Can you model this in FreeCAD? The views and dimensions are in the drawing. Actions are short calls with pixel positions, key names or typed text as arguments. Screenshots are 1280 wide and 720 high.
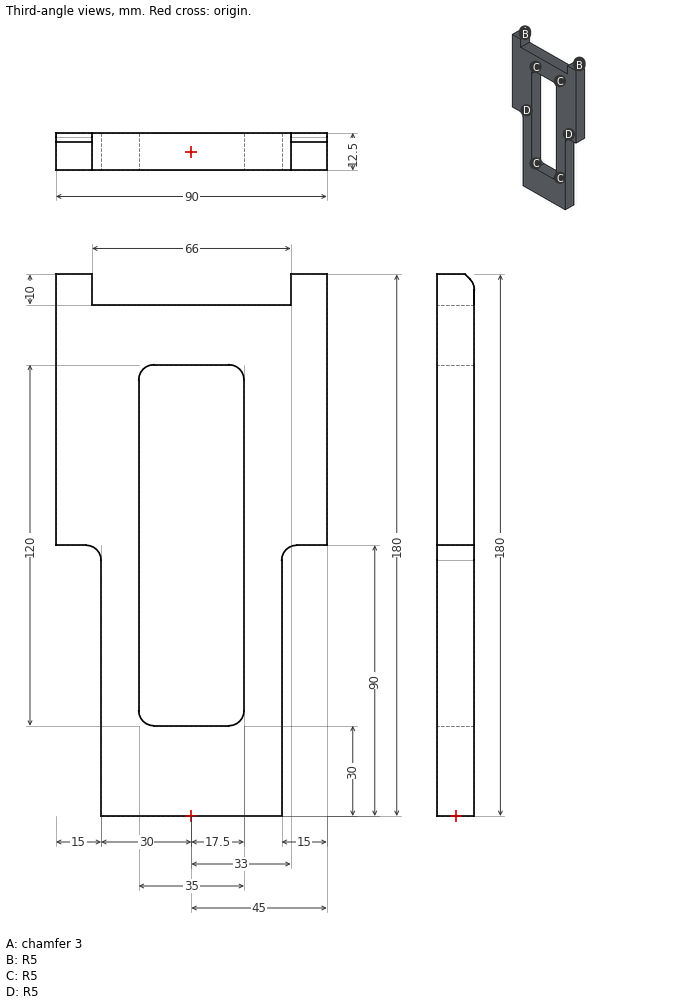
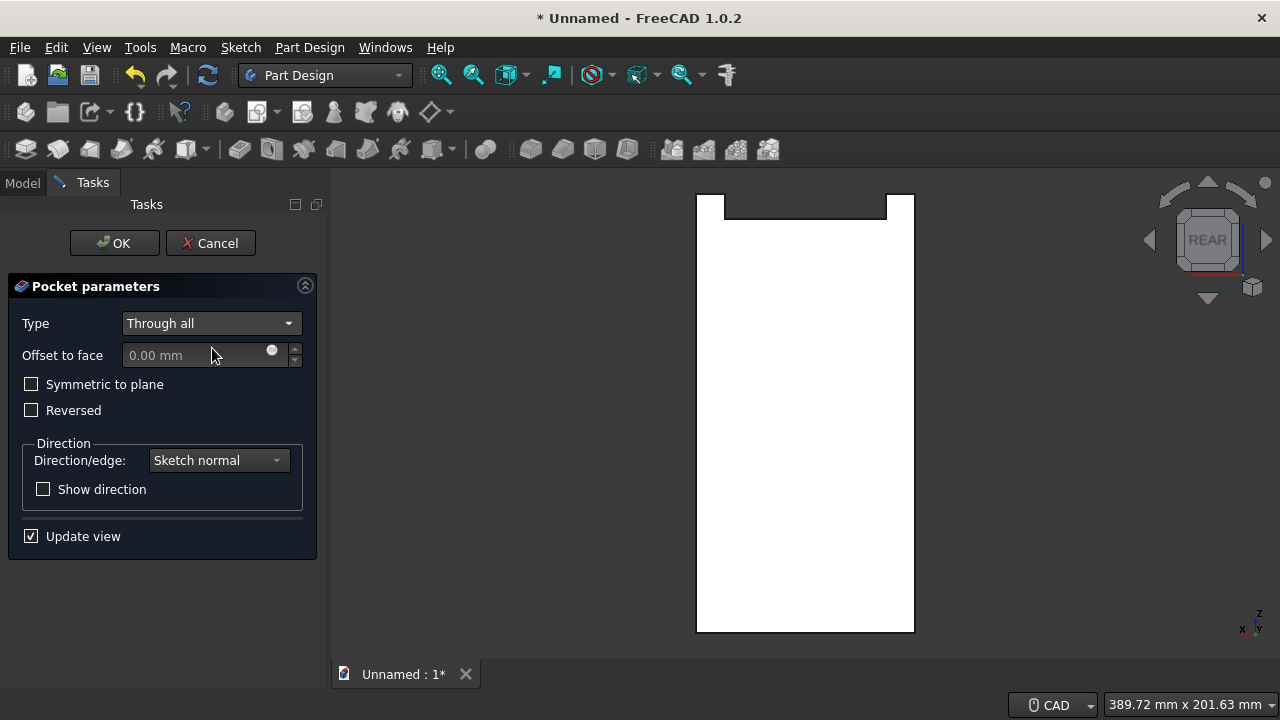
click(115, 243)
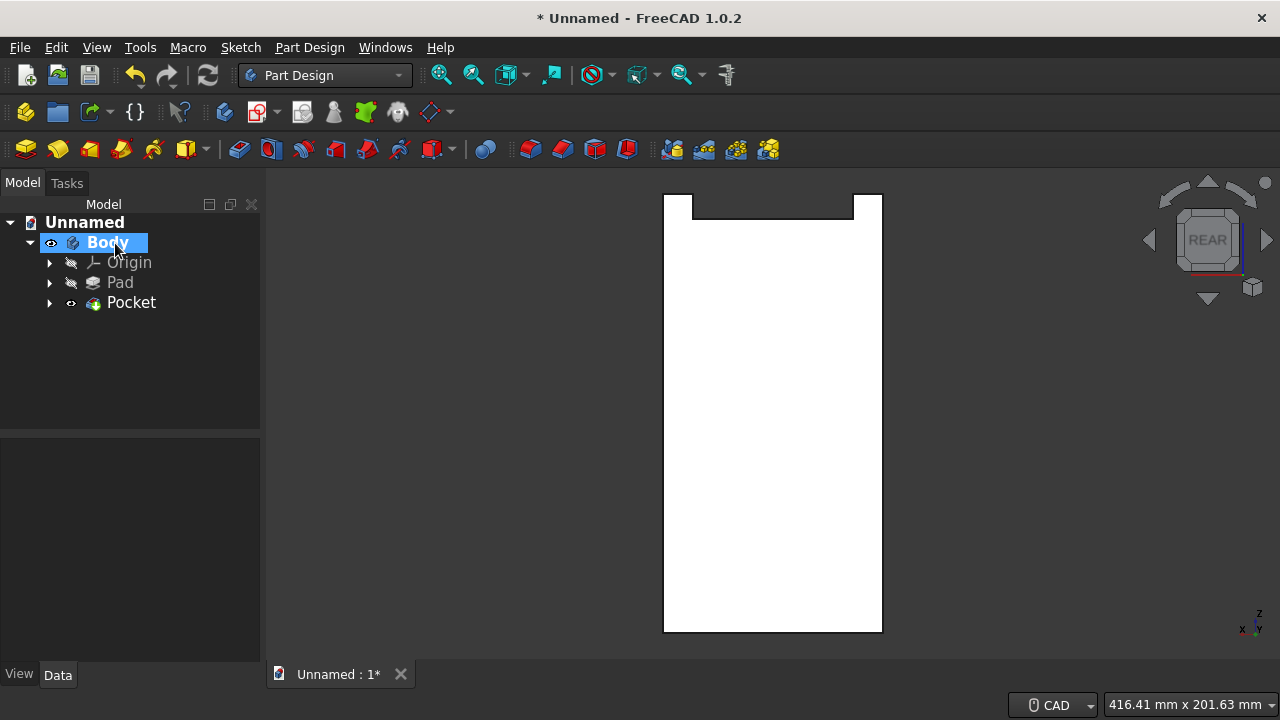
key(0)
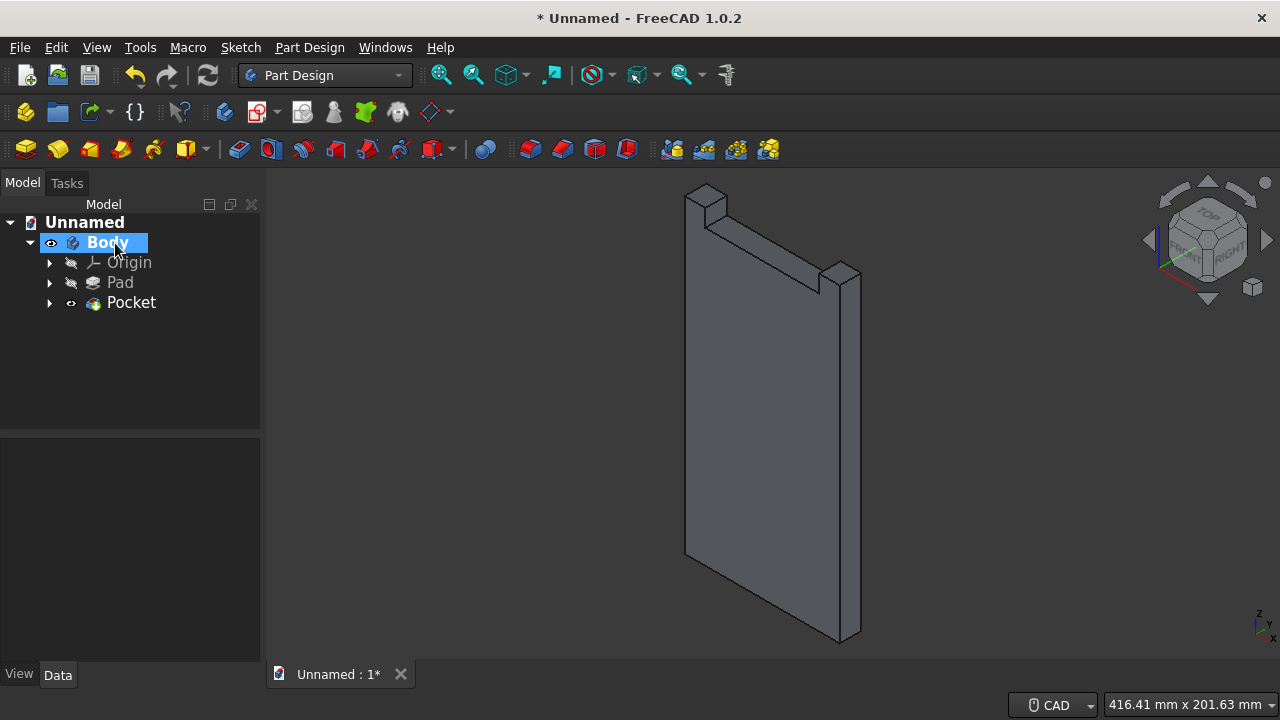
key(2)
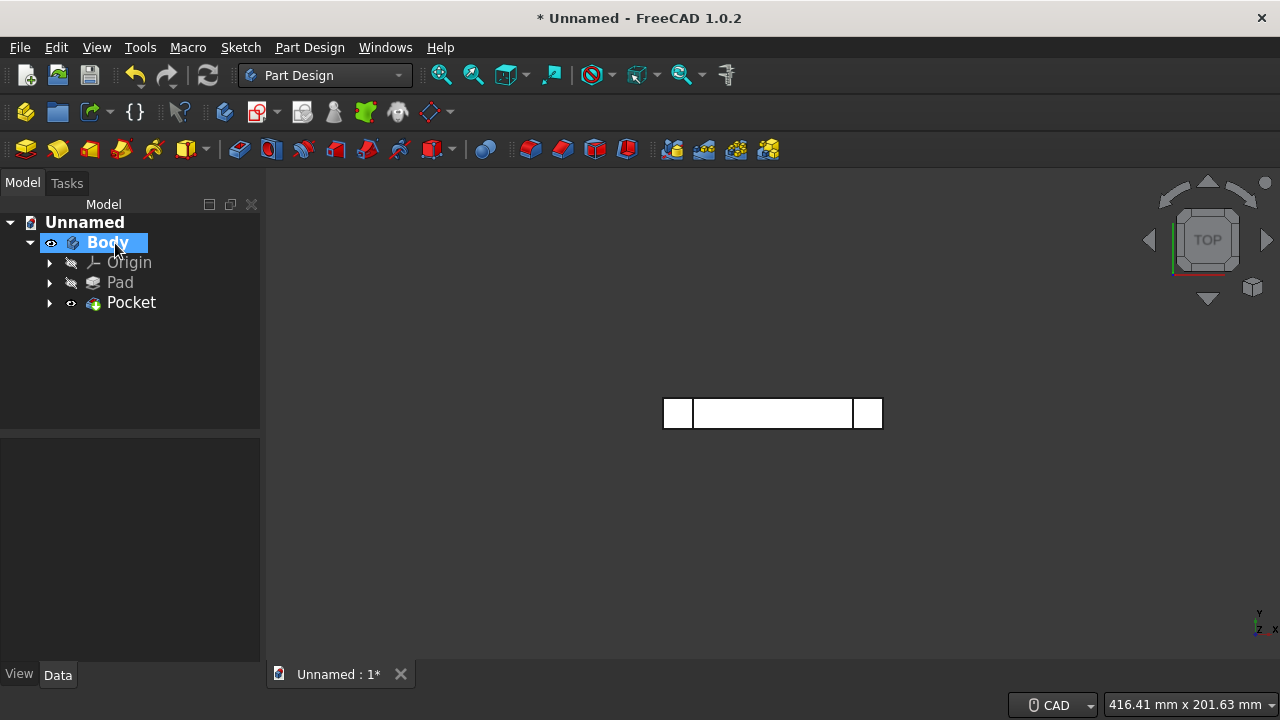
click(442, 76)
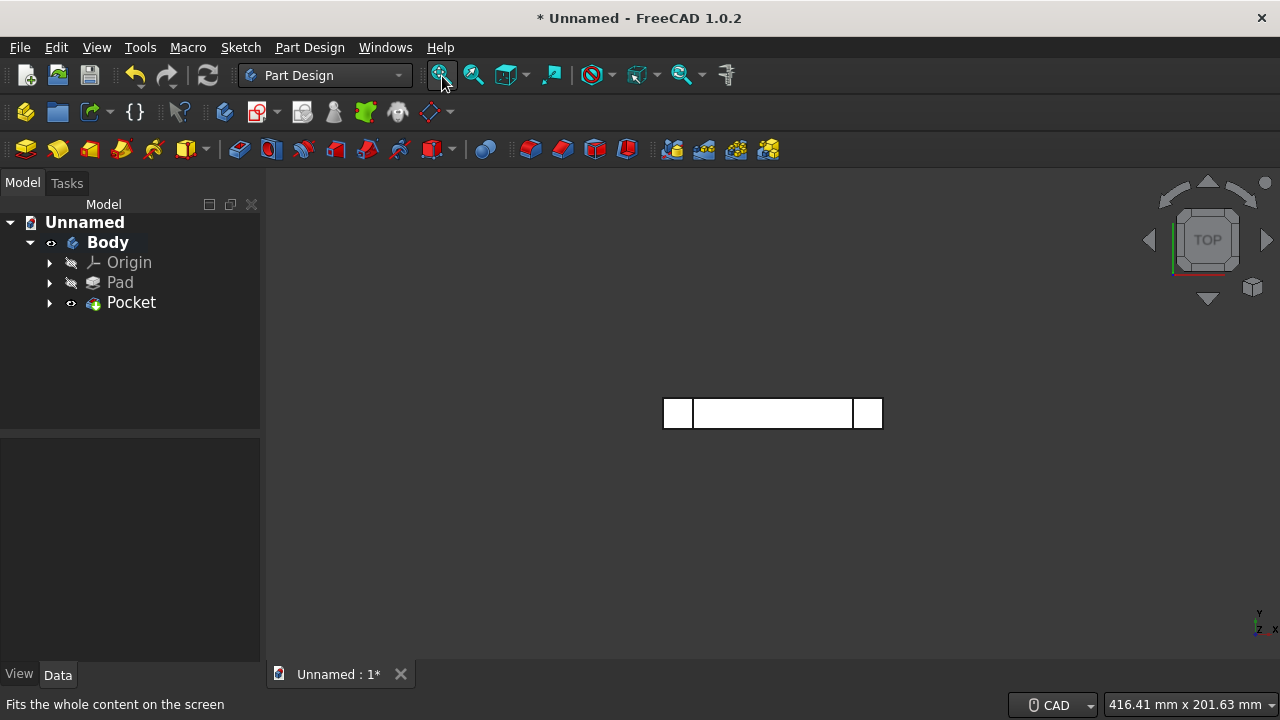
click(868, 397)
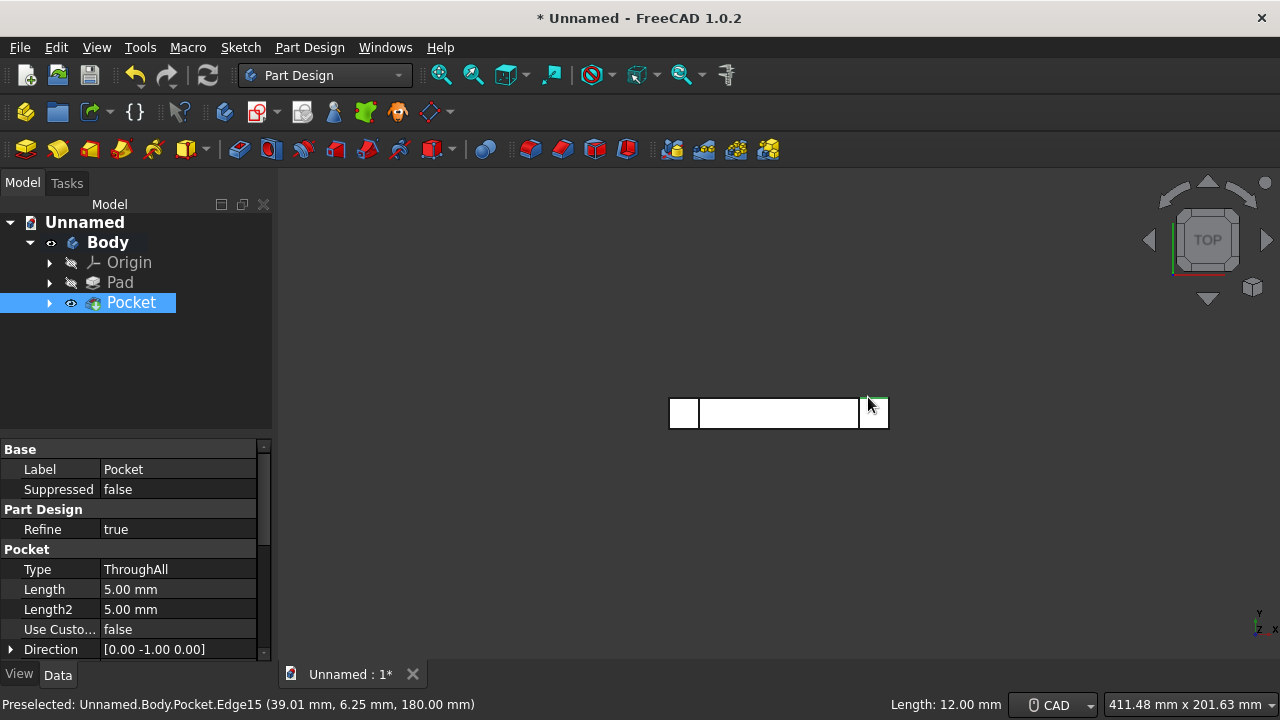
click(684, 397, ctrl)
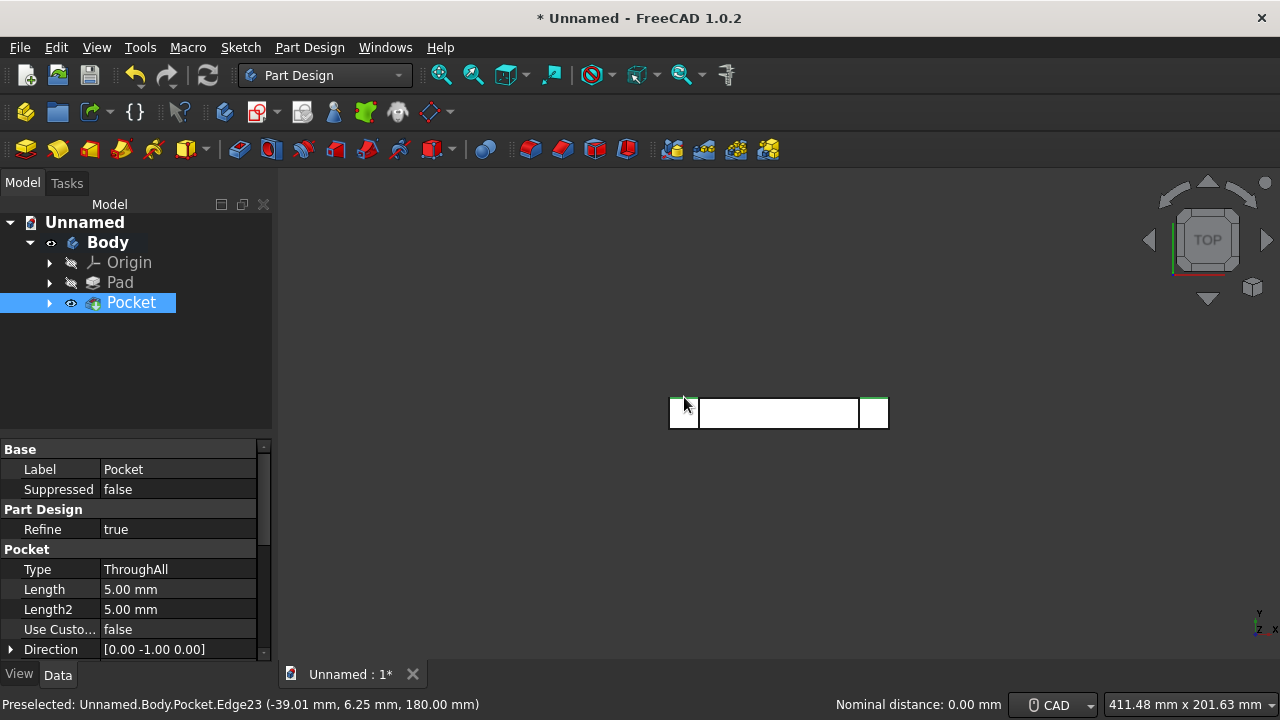
click(564, 150)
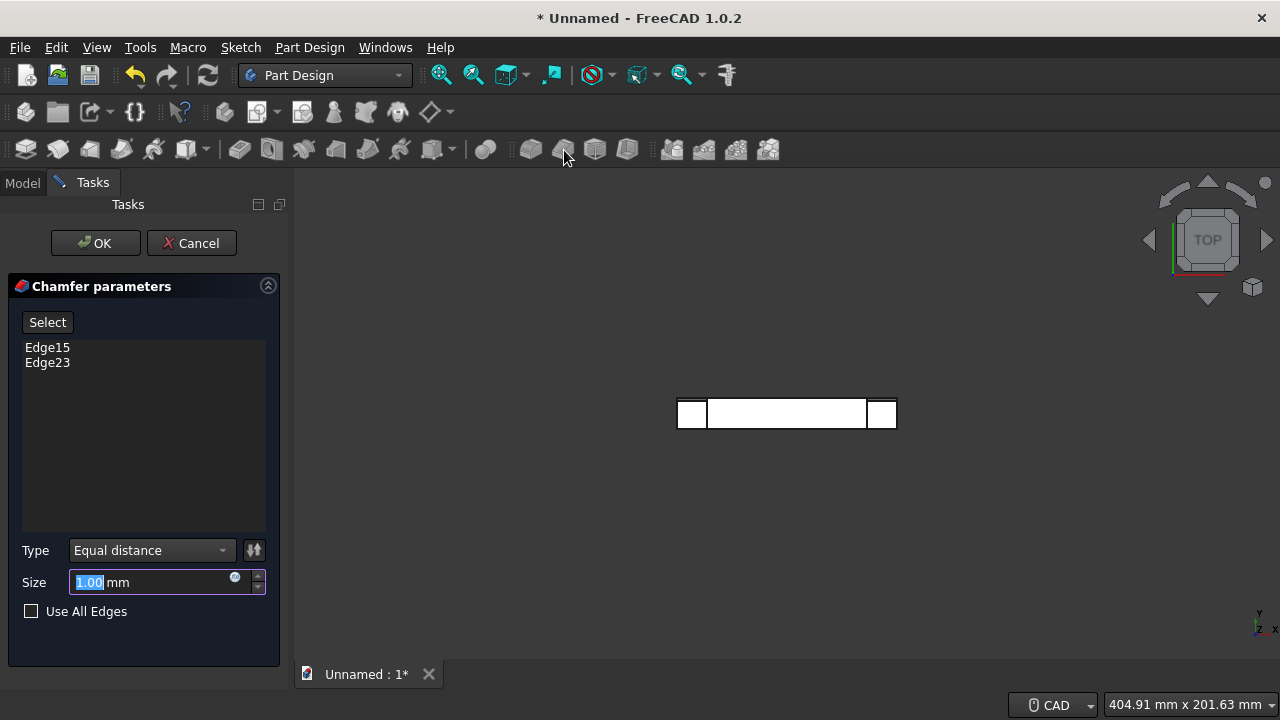
text(3)
key(Tab)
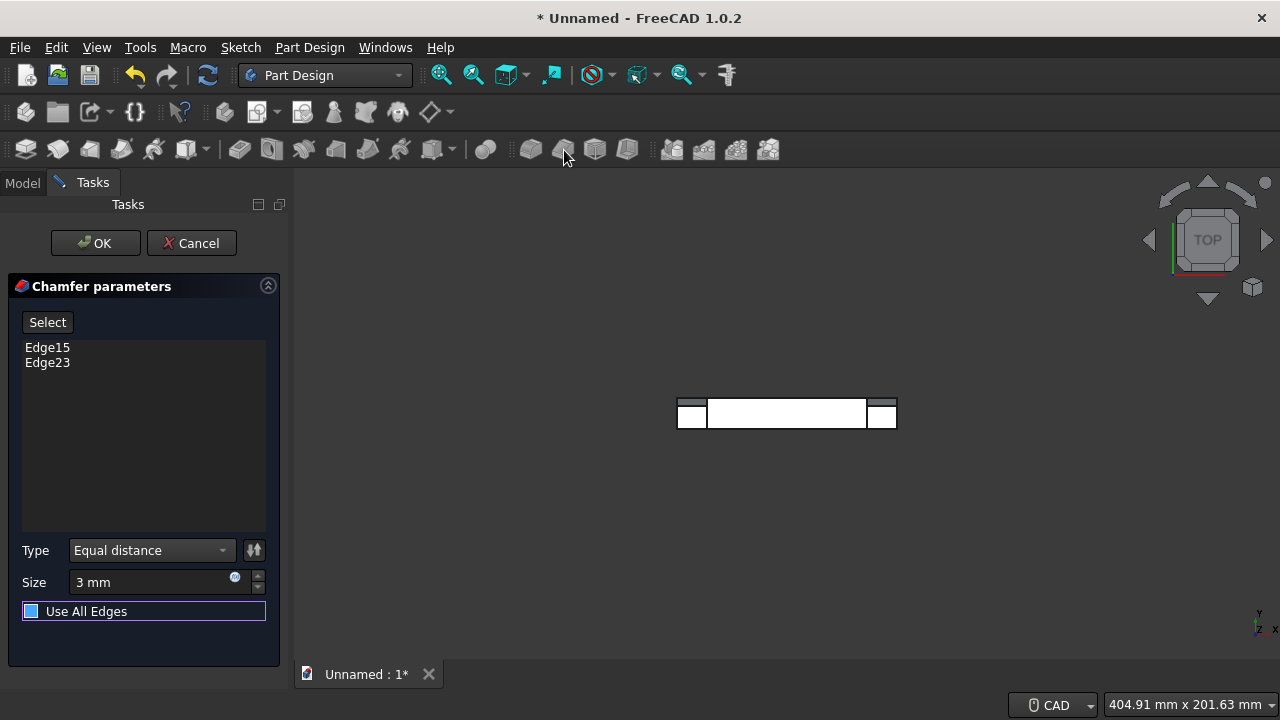
click(96, 243)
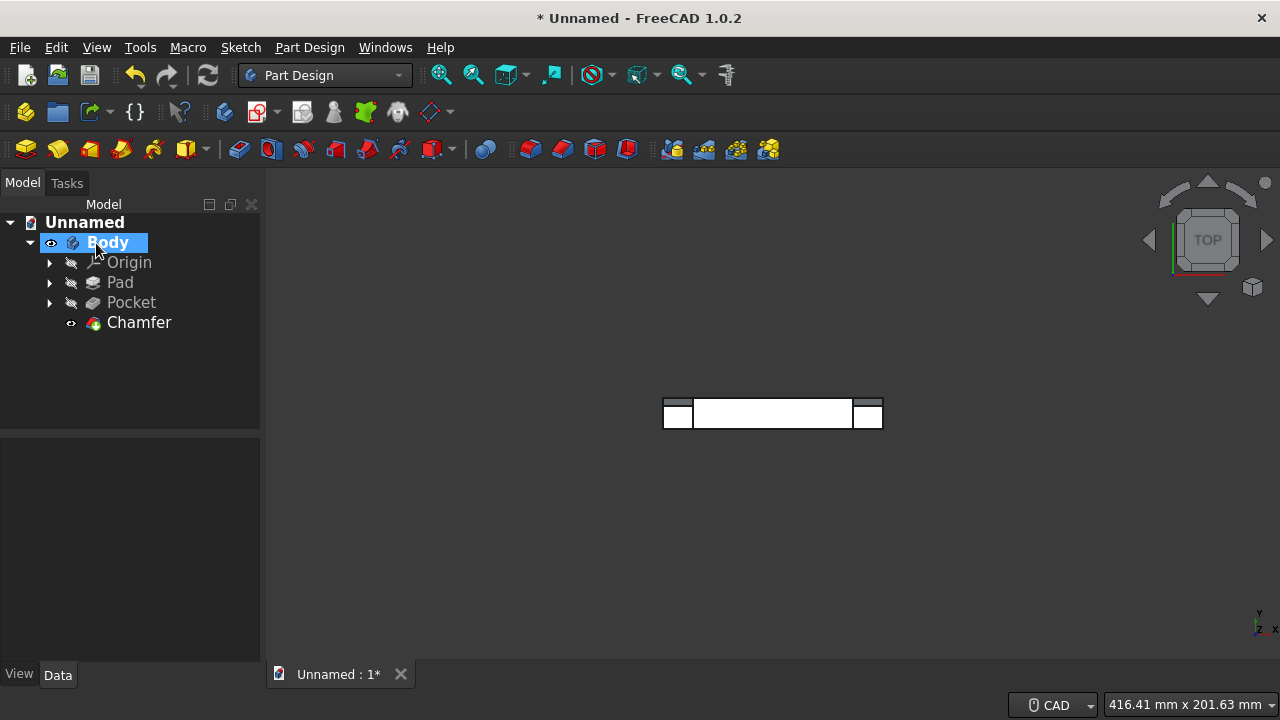
click(442, 76)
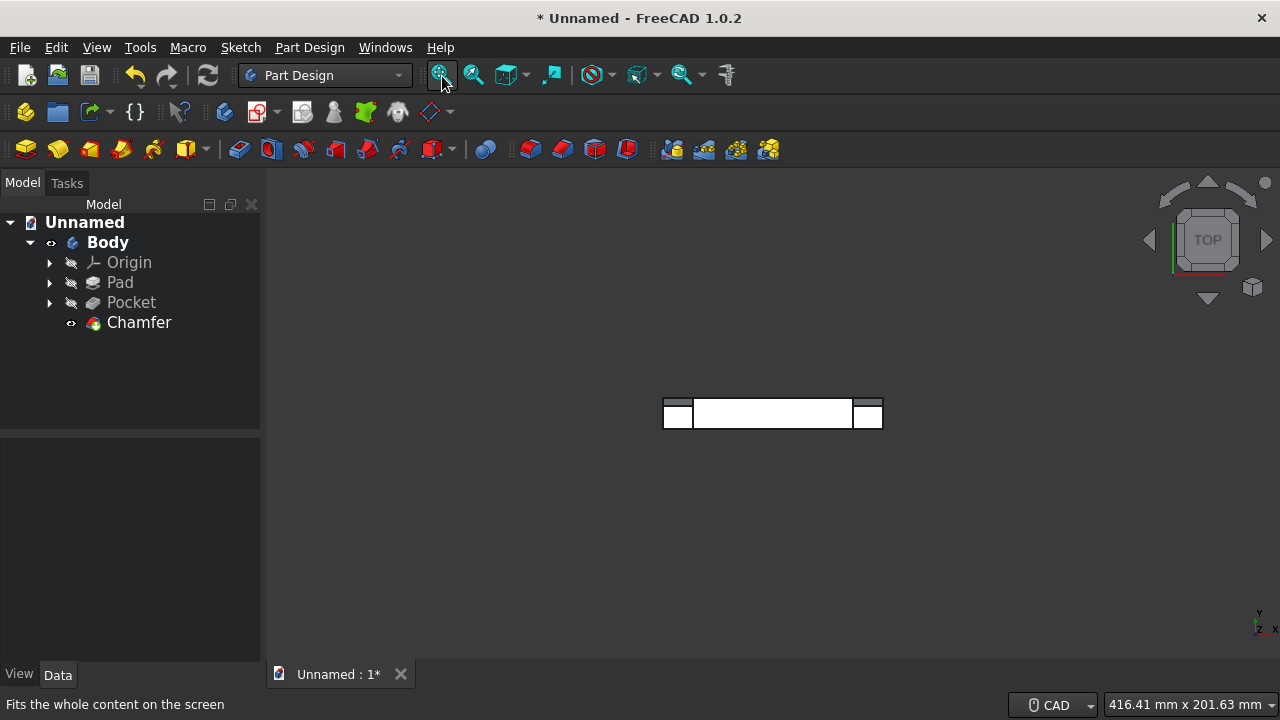
key(0)